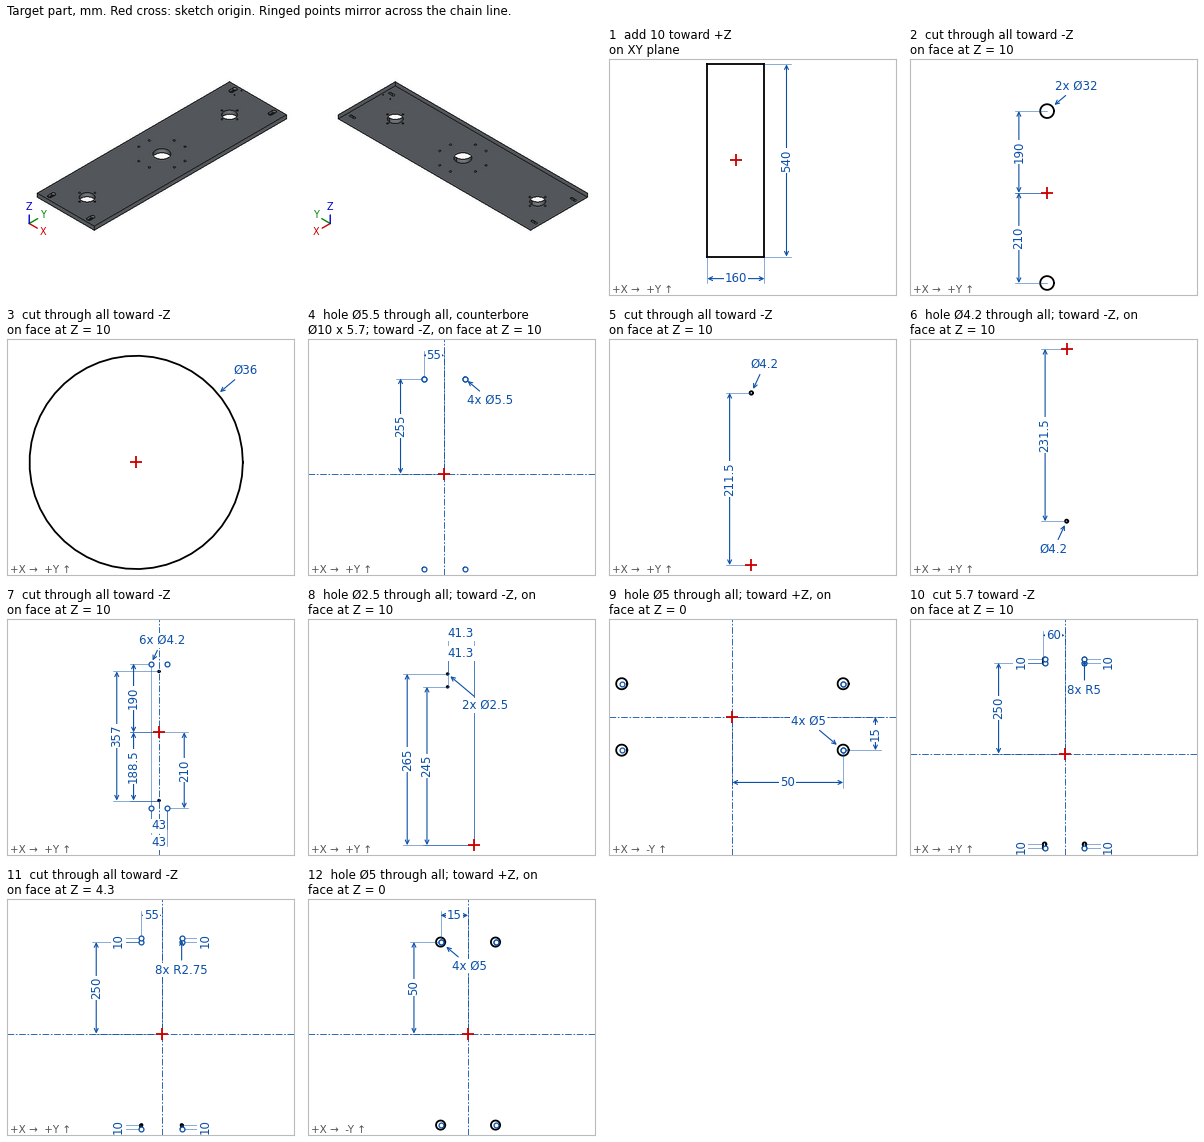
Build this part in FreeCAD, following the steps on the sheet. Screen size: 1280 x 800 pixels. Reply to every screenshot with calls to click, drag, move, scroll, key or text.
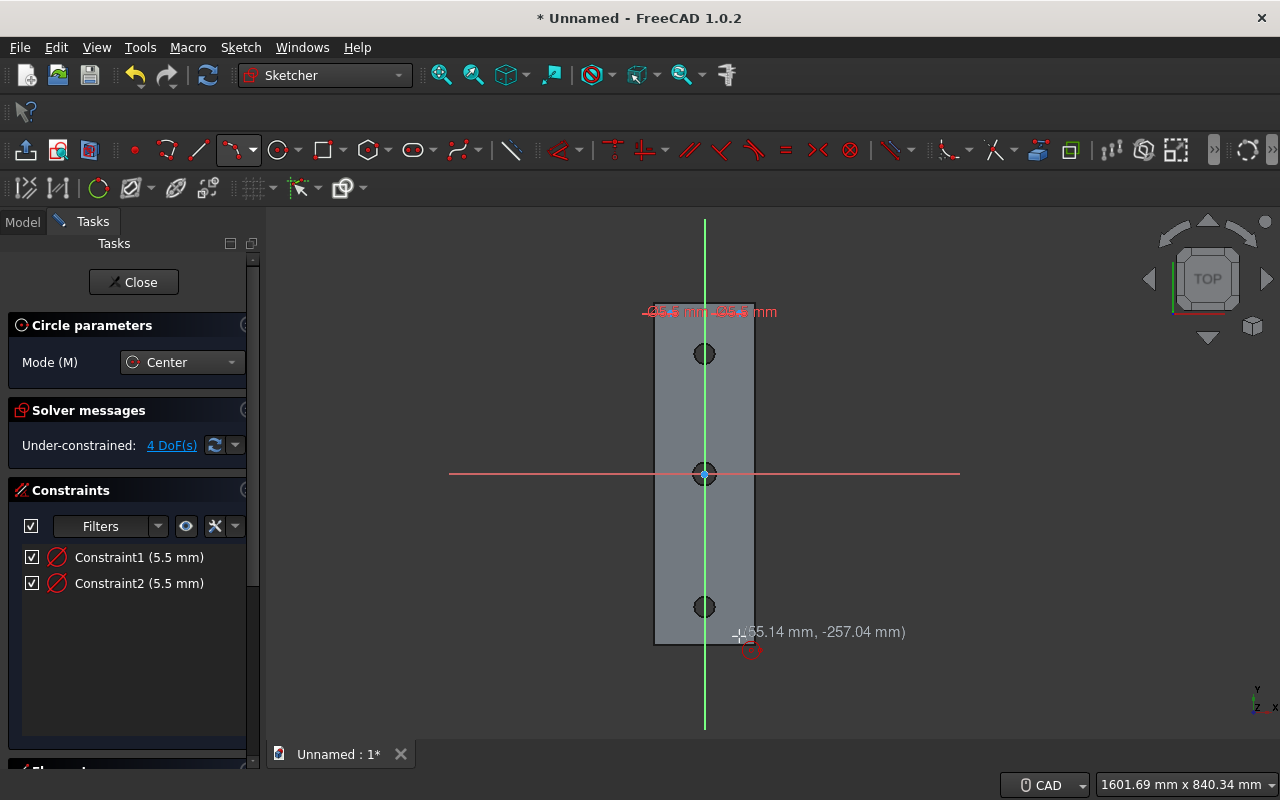
click(739, 636)
move(741, 634)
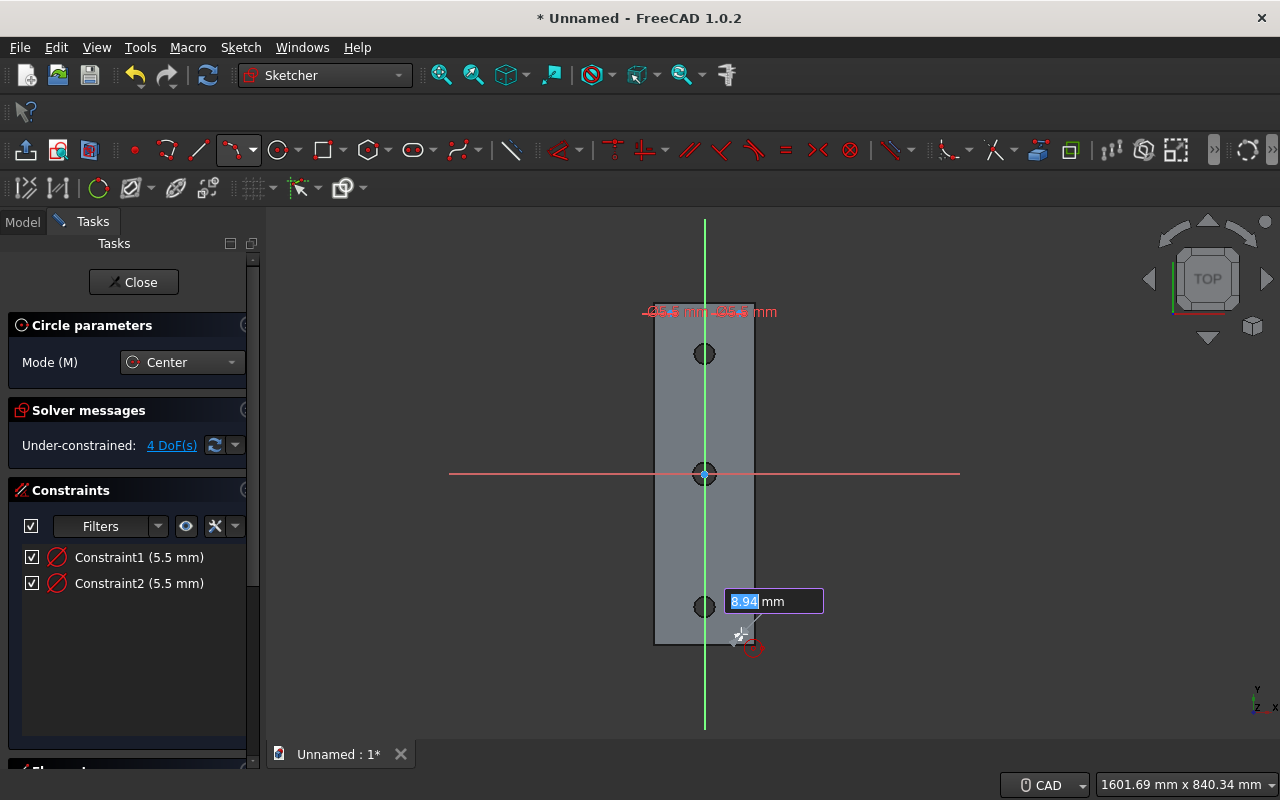
text(5.5)
key(Return)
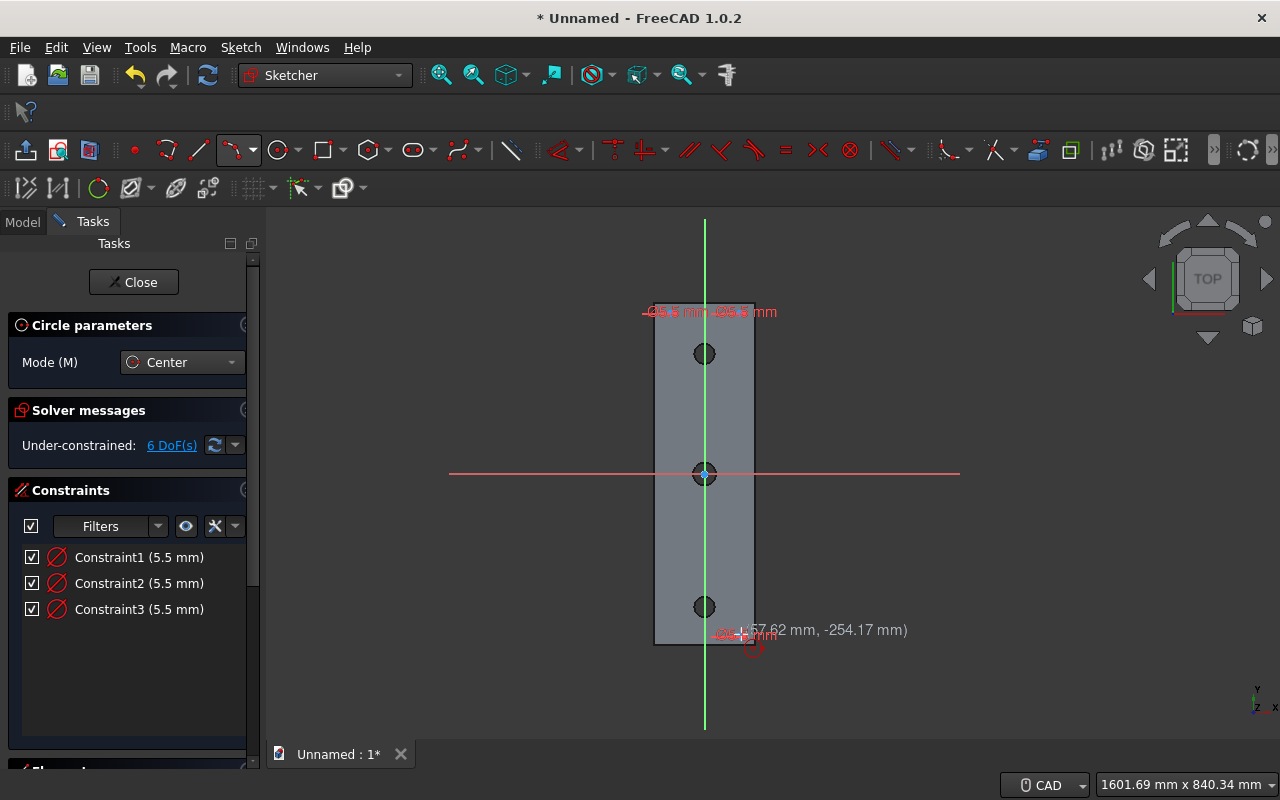
scroll(670, 636, up, 13)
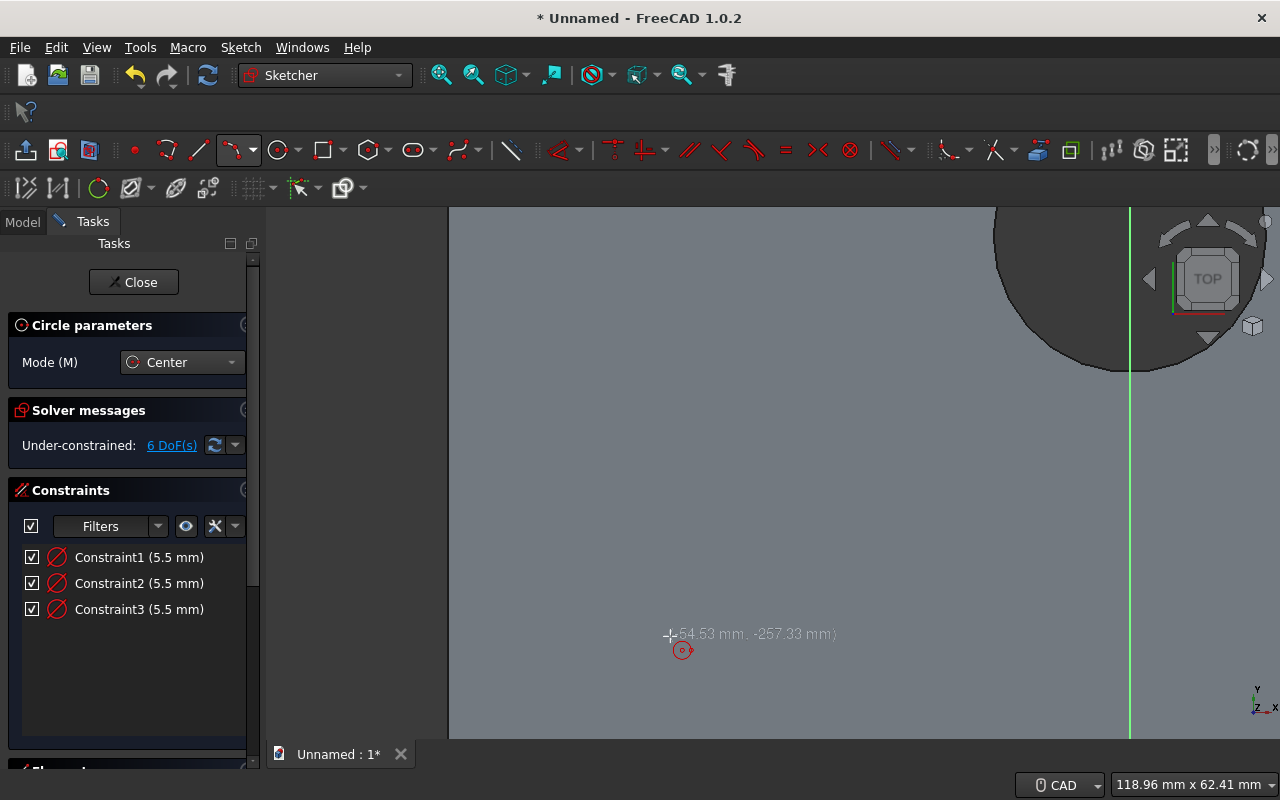
scroll(670, 636, down, 13)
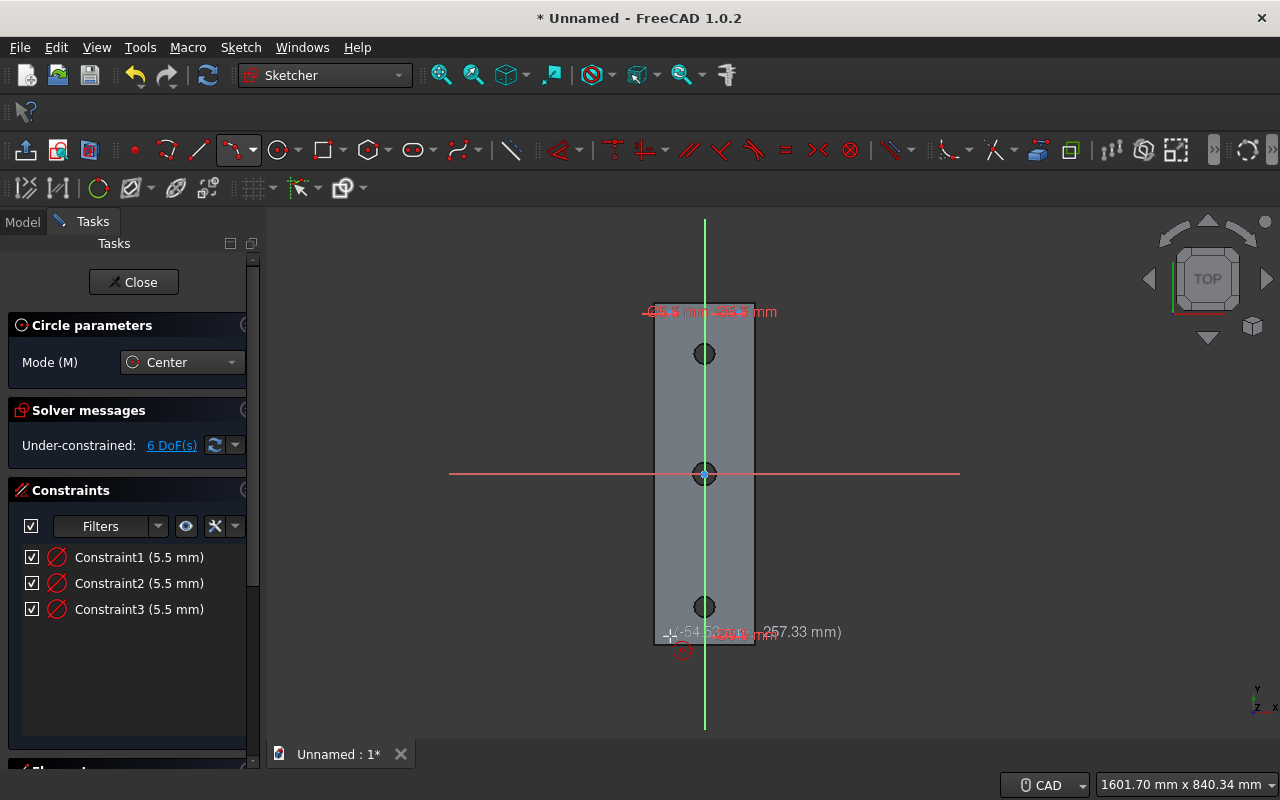
click(670, 636)
move(671, 634)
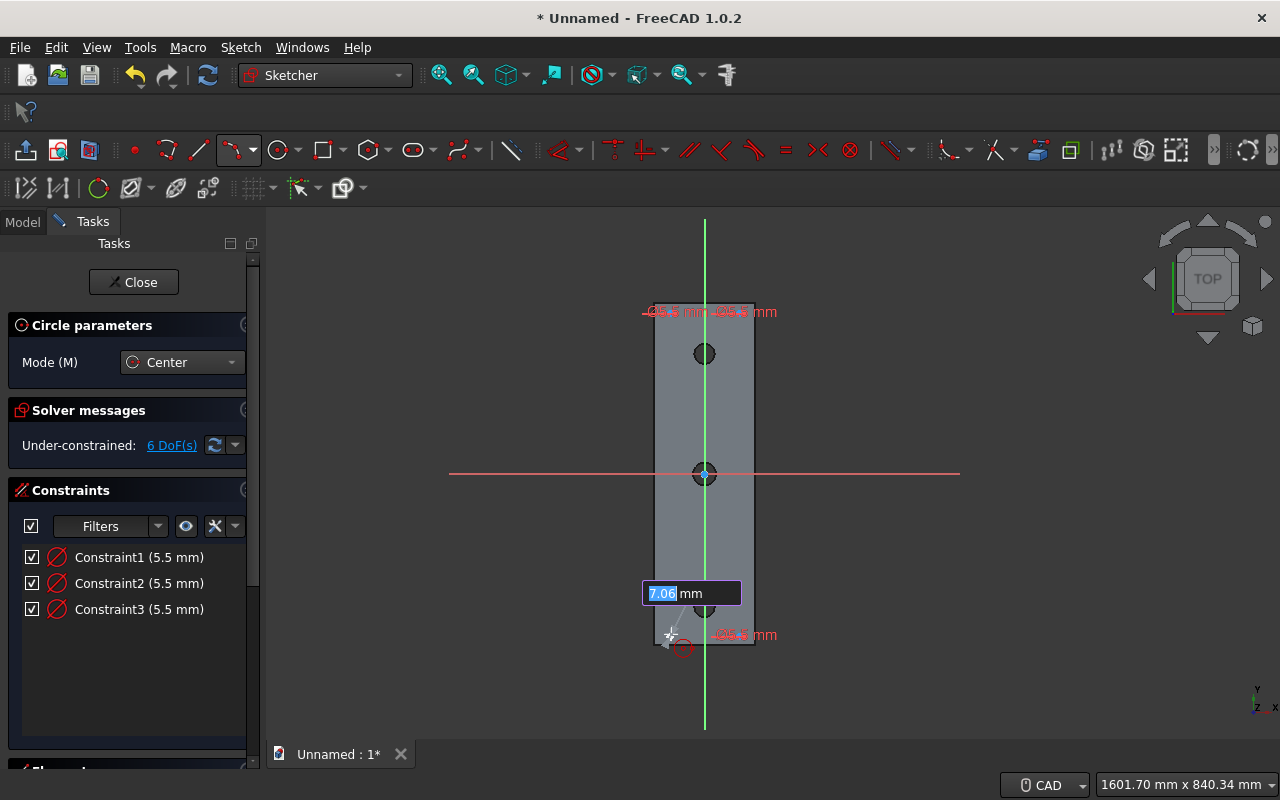
text(5.5)
key(Return)
key(Escape)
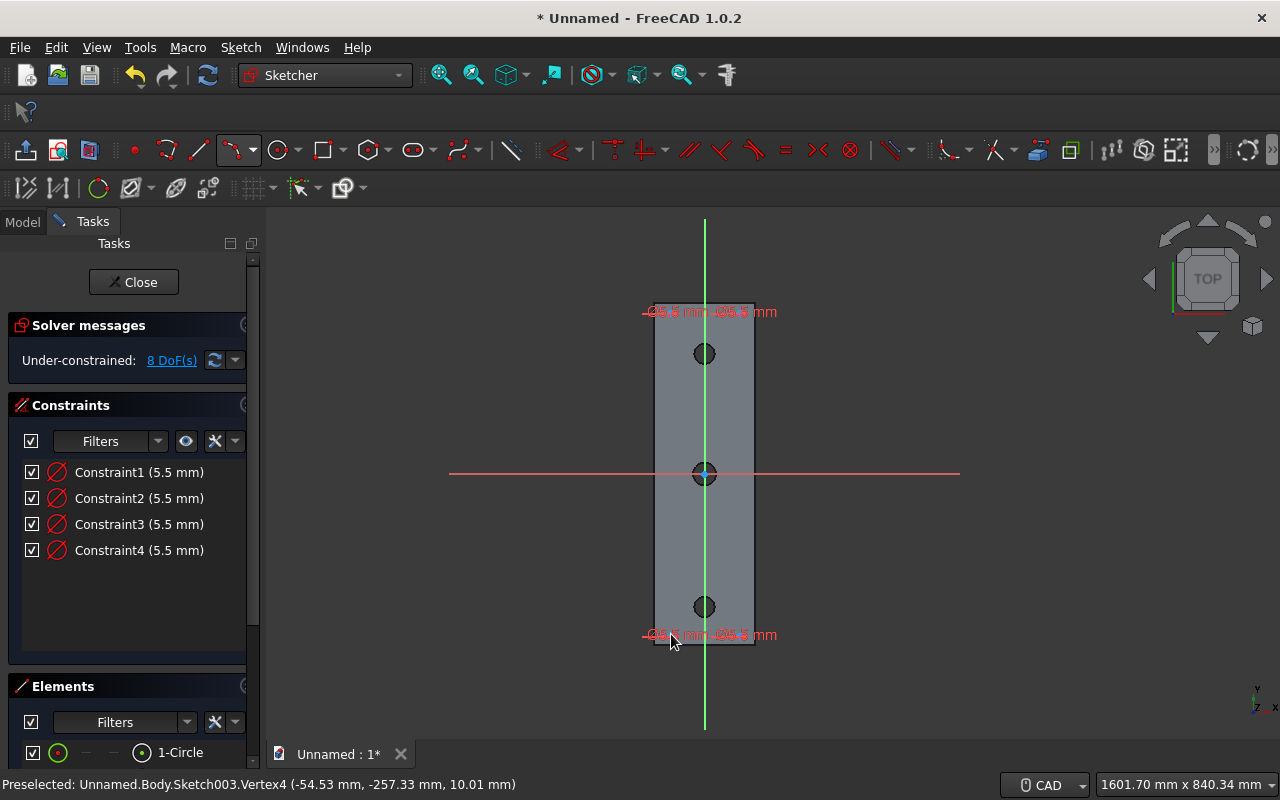
click(670, 314)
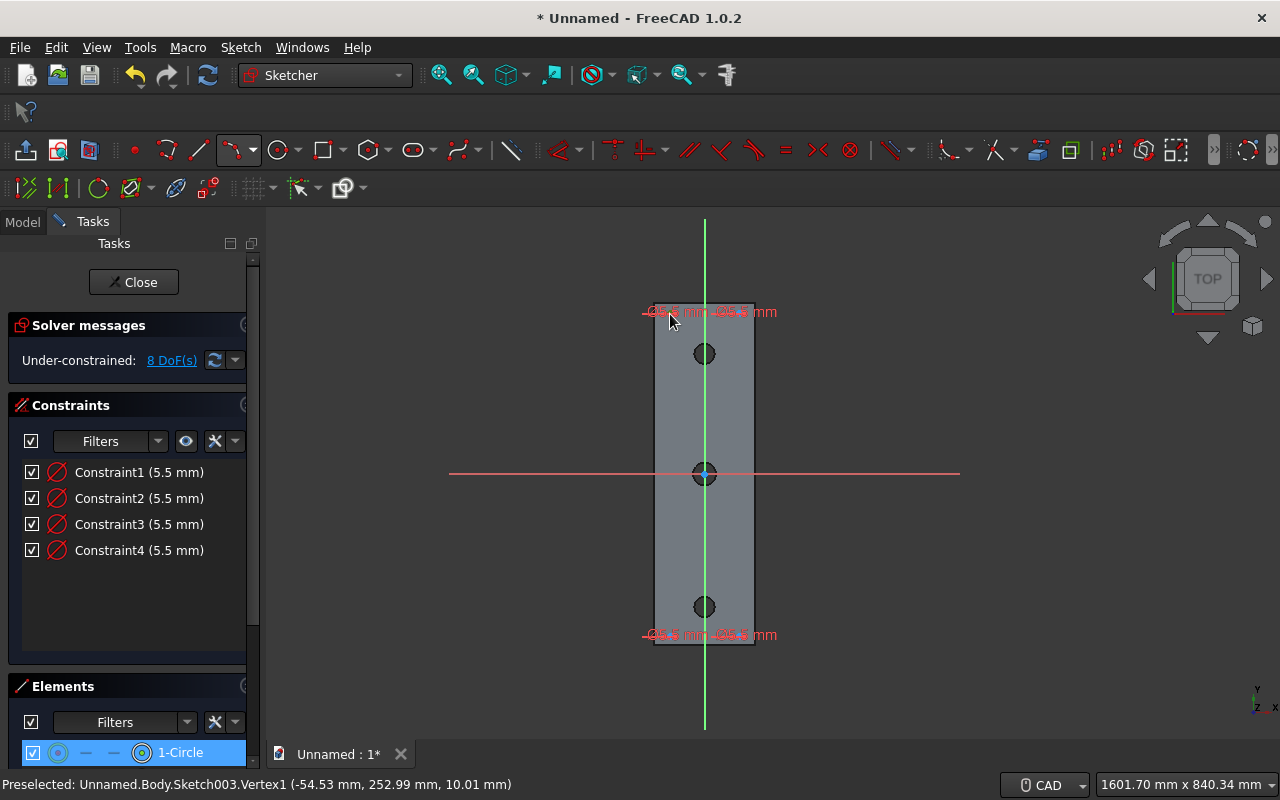
click(739, 314)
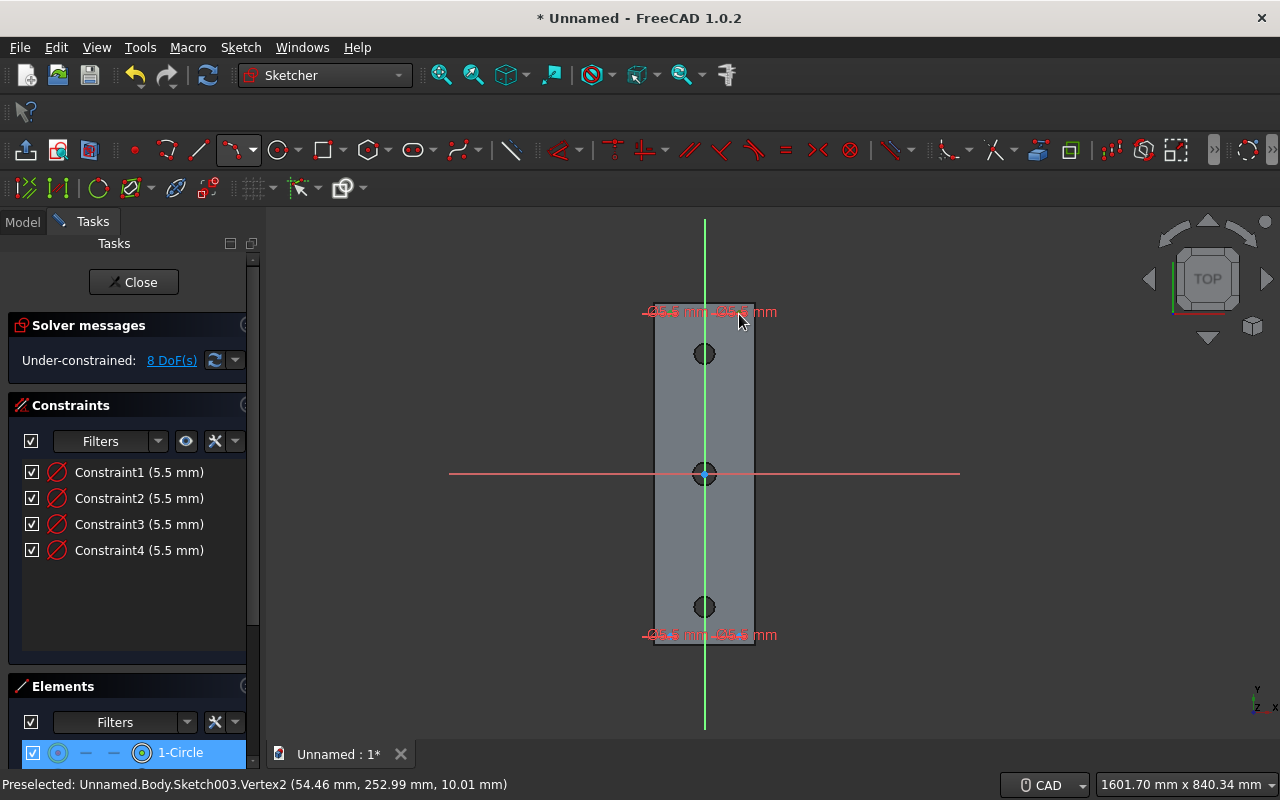
click(705, 677)